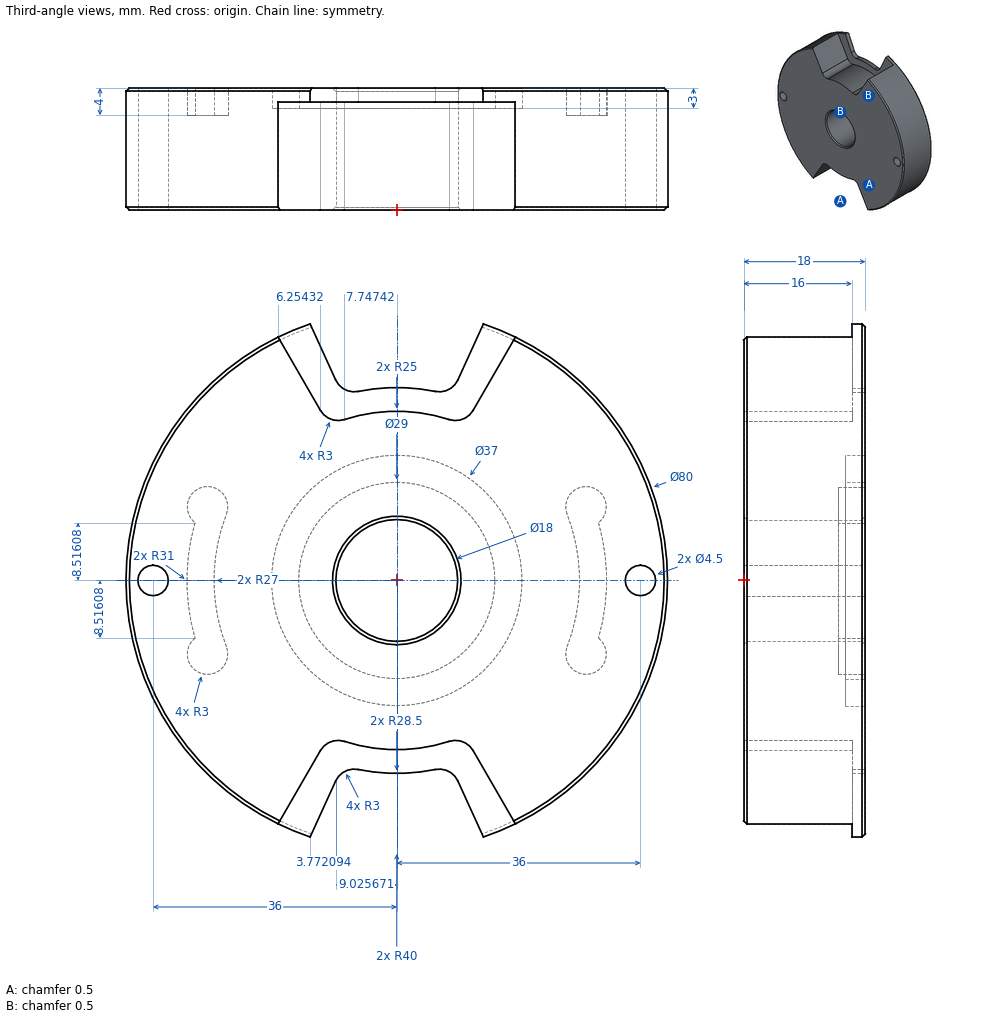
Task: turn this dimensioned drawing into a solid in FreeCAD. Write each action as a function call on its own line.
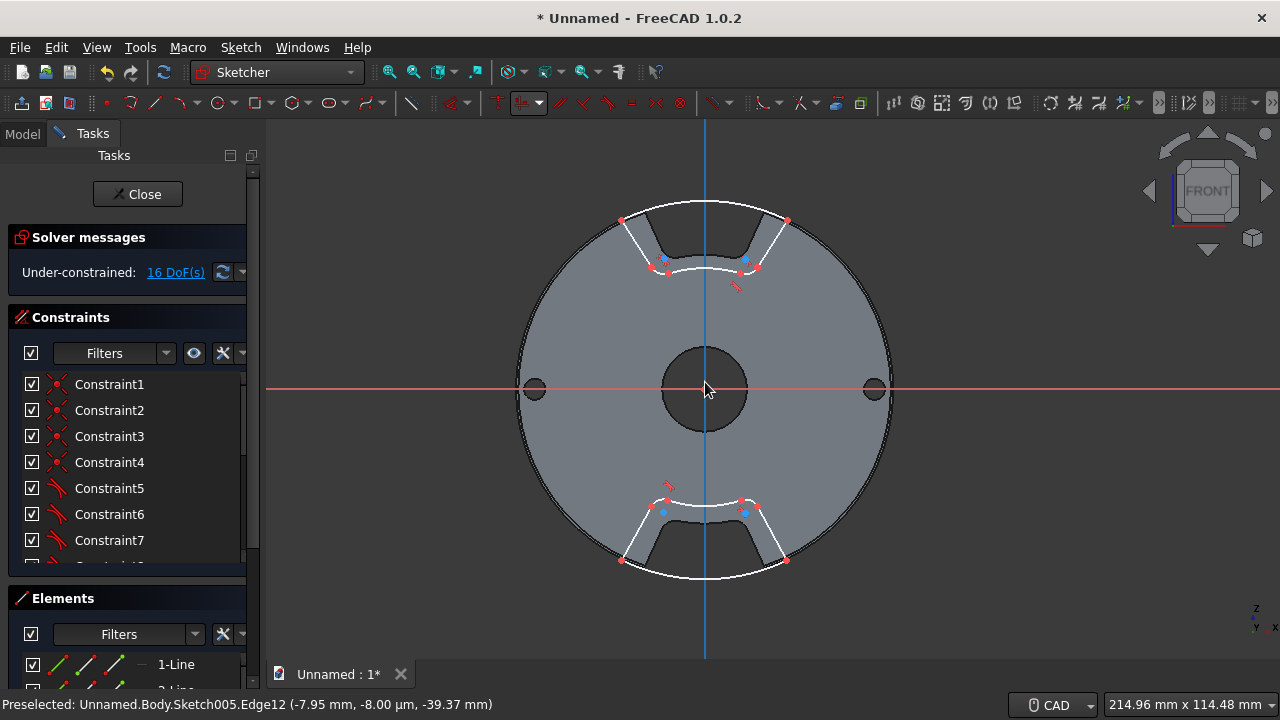
scroll(656, 271, up, 5)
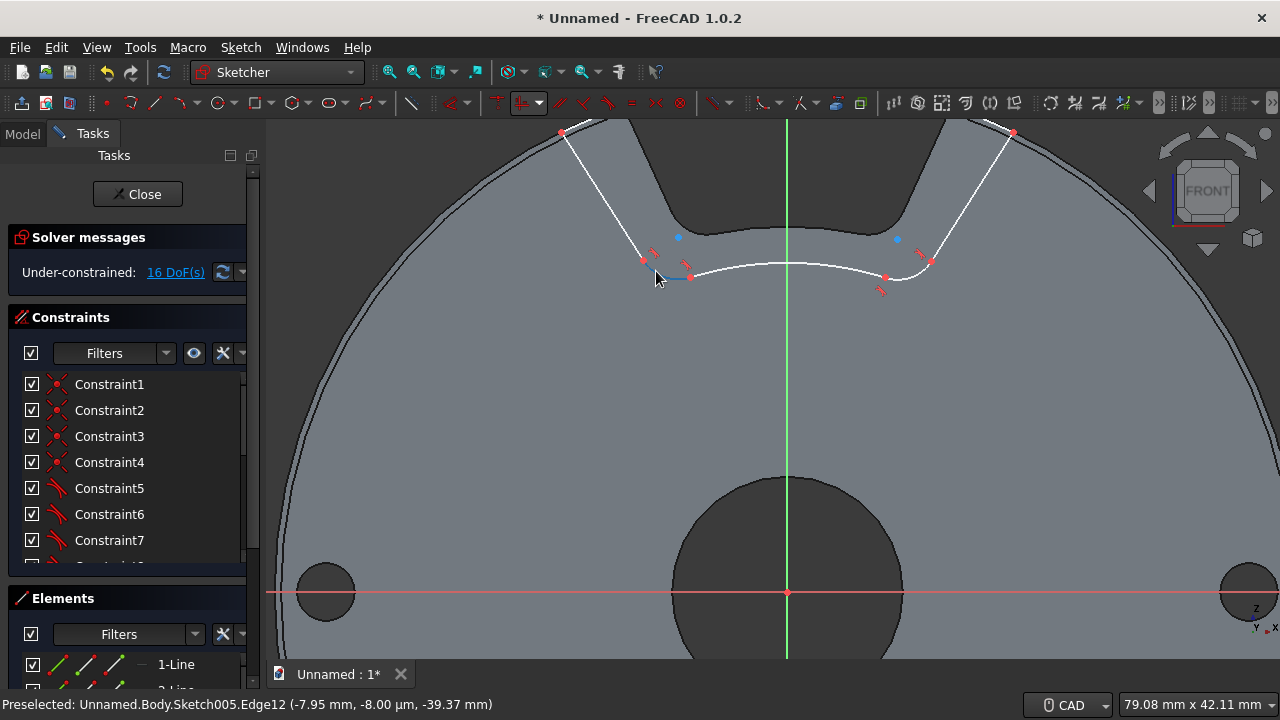
click(654, 272)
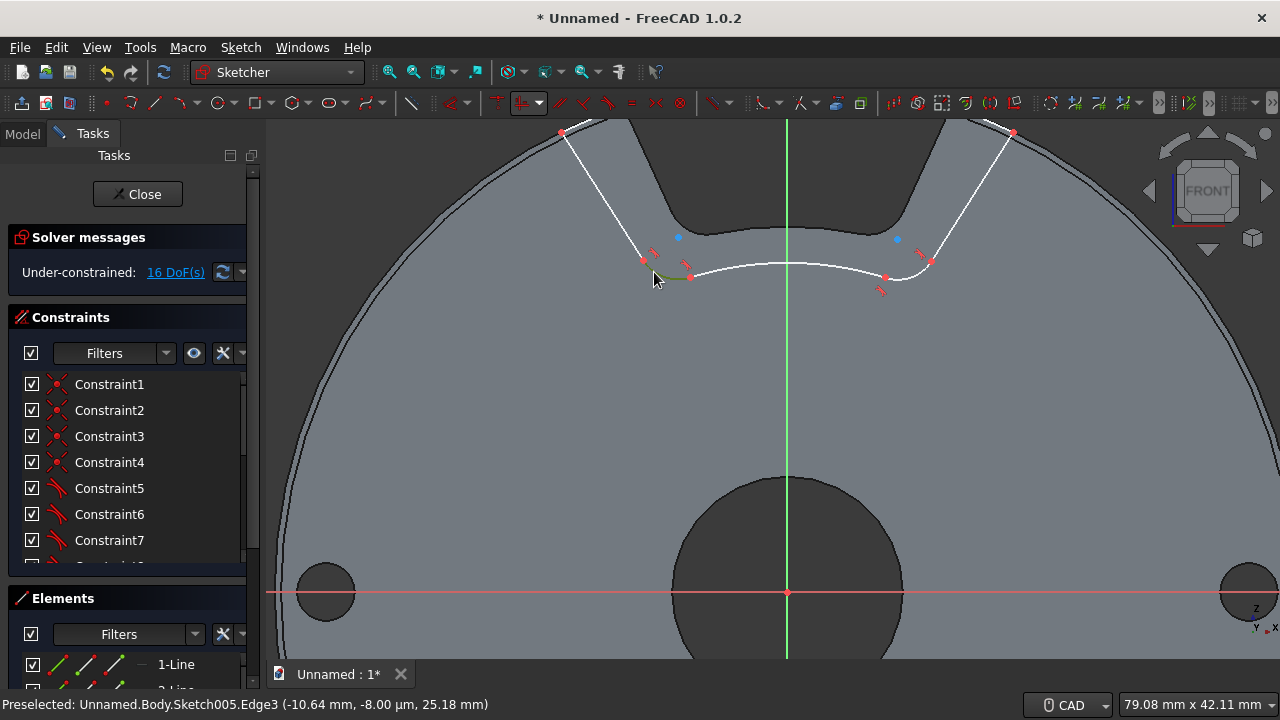
click(901, 280)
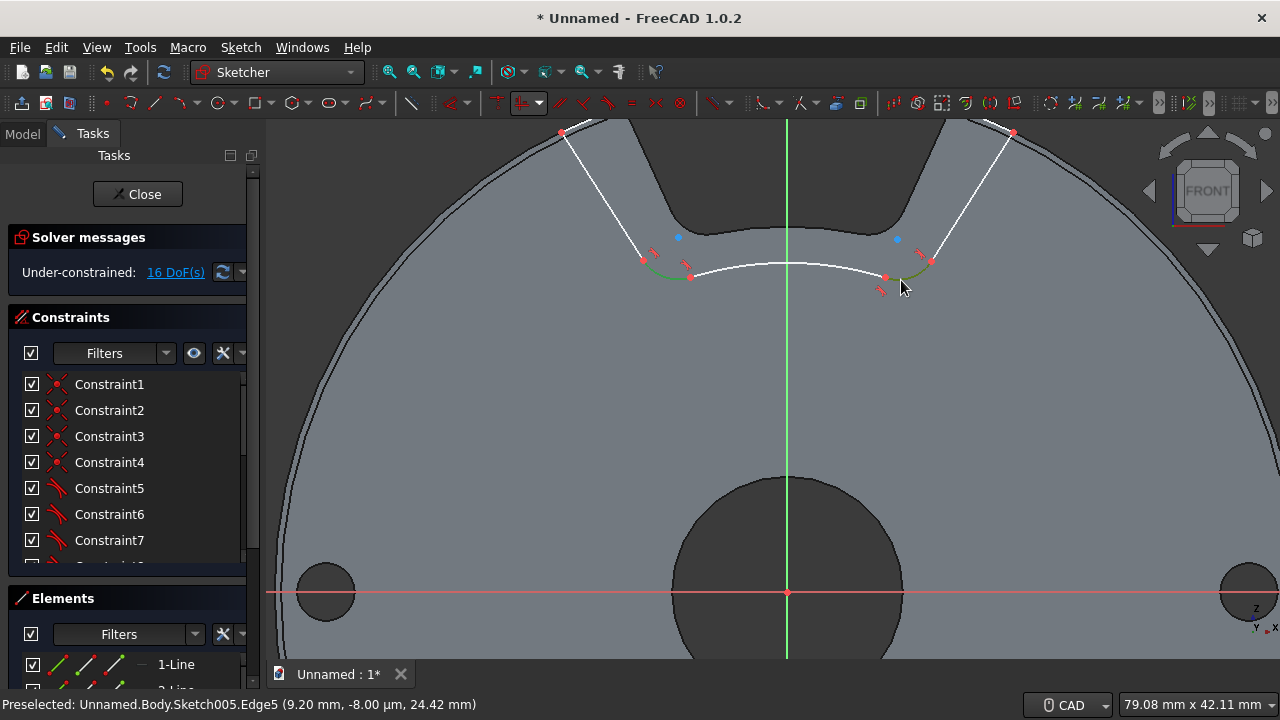
scroll(656, 271, down, 5)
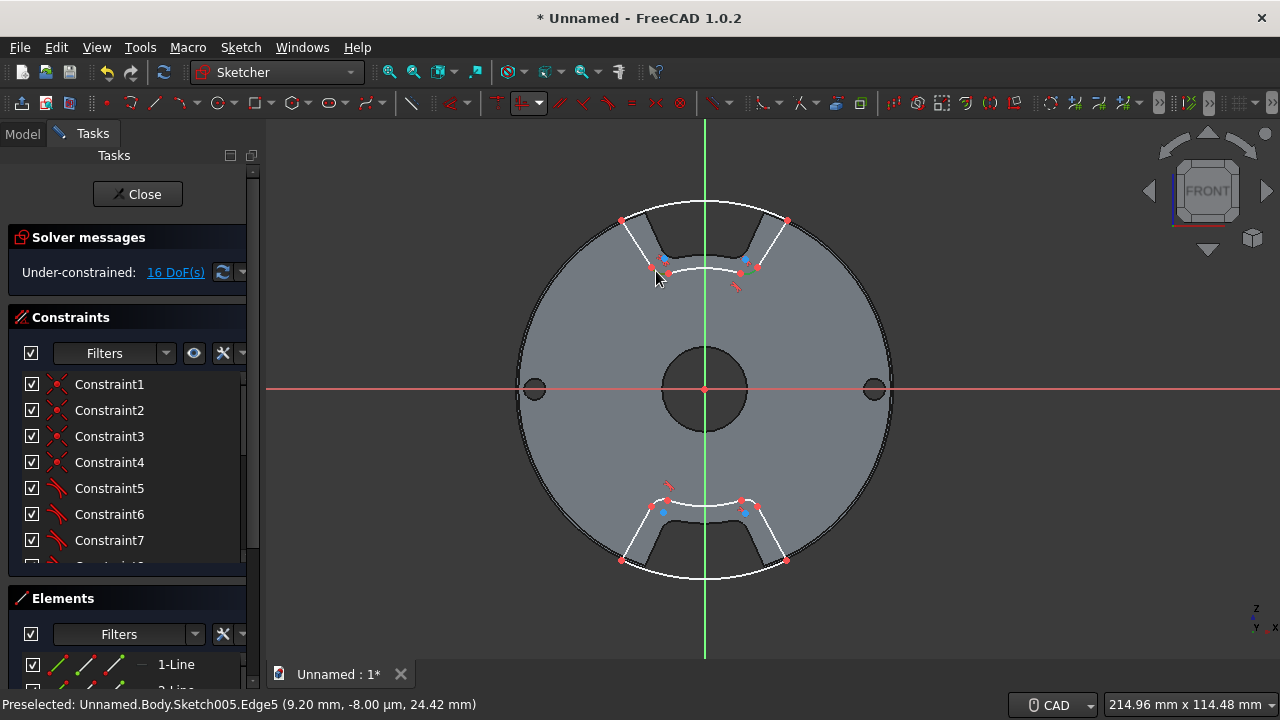
scroll(754, 502, up, 5)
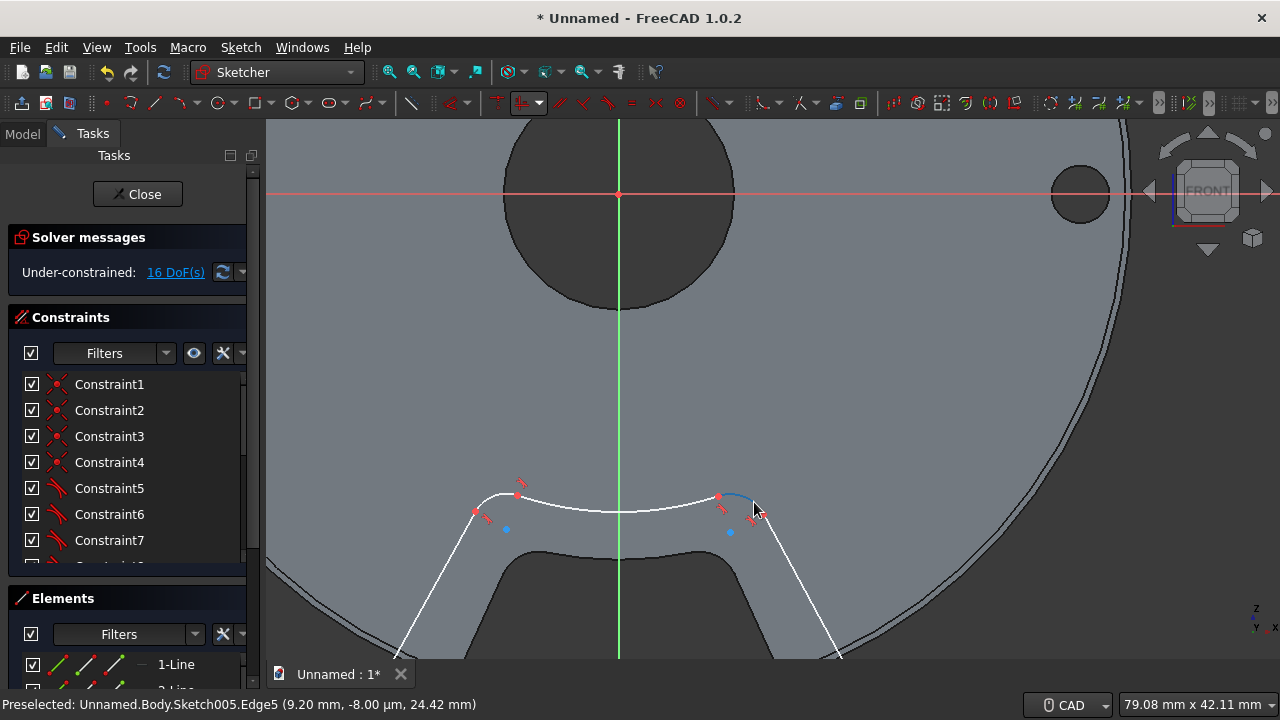
click(753, 502)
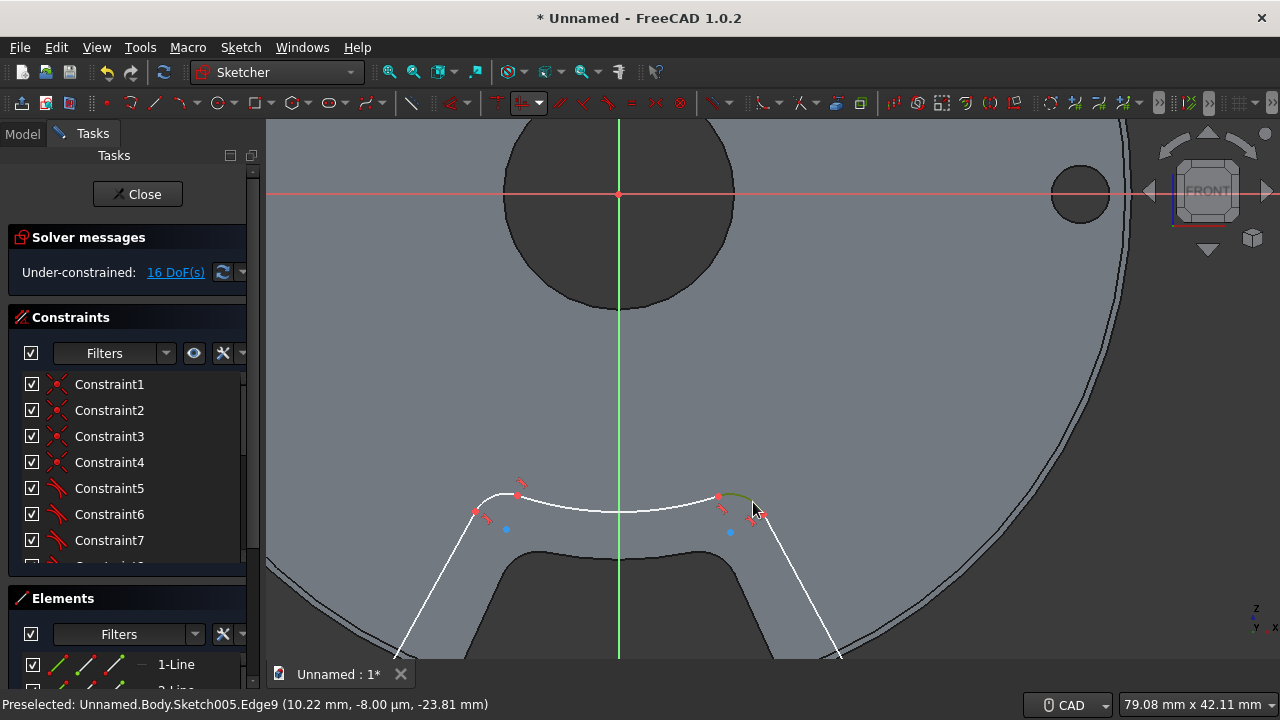
click(503, 494)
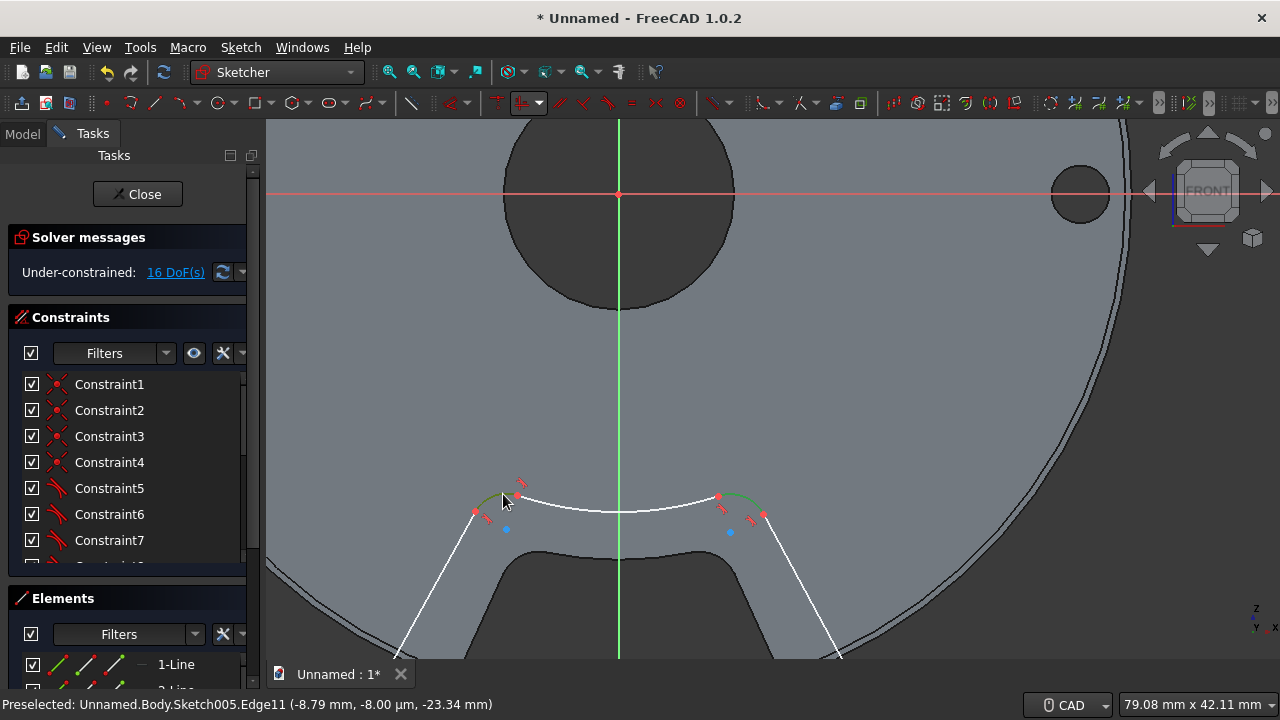
click(632, 104)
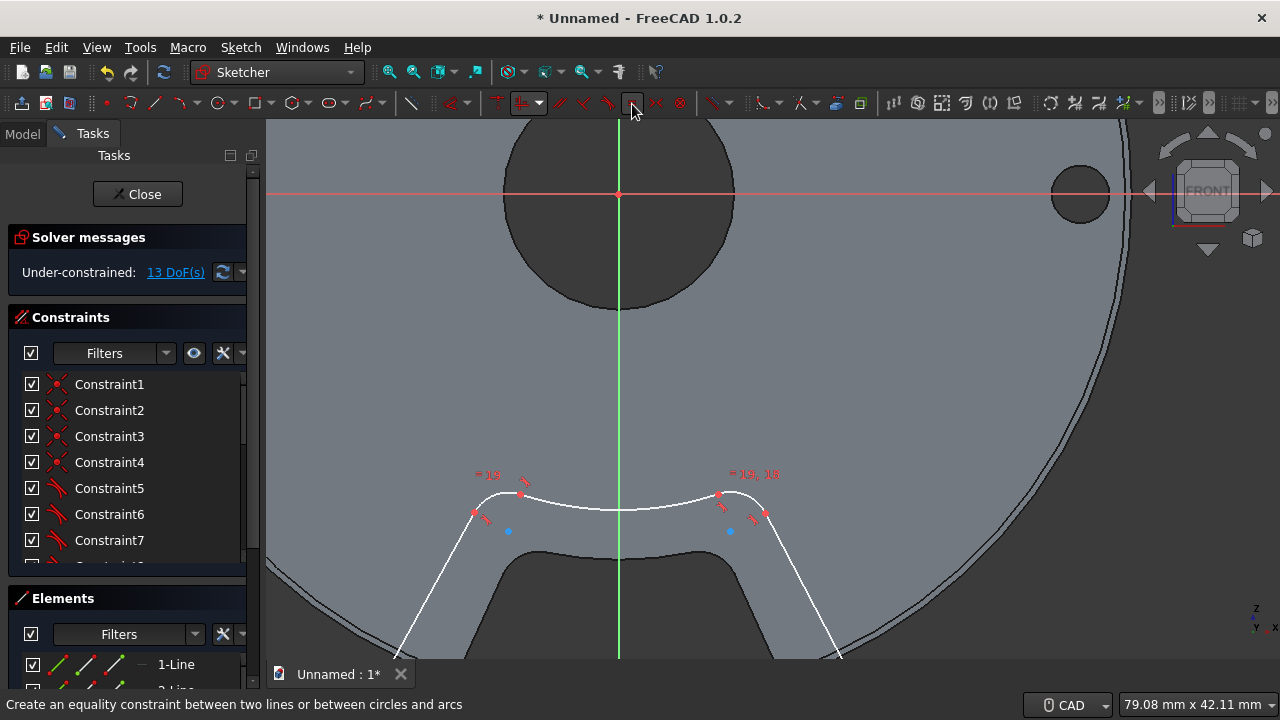
scroll(754, 502, down, 5)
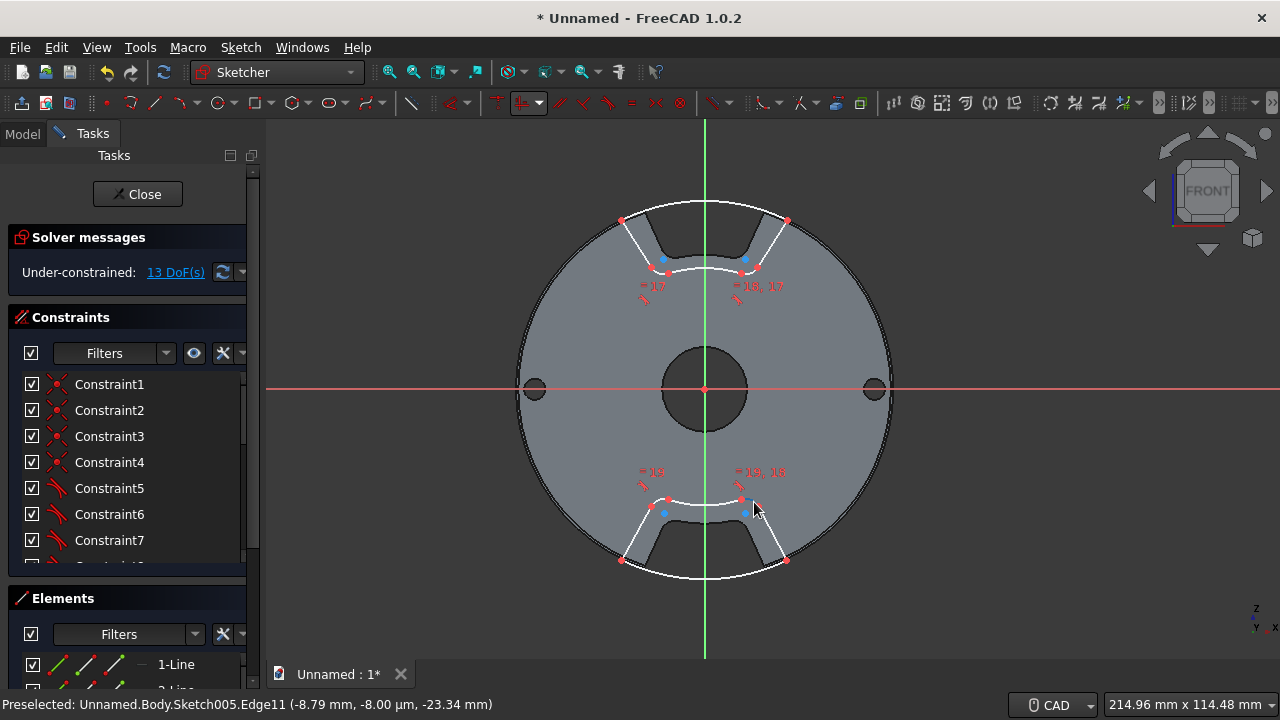
click(719, 269)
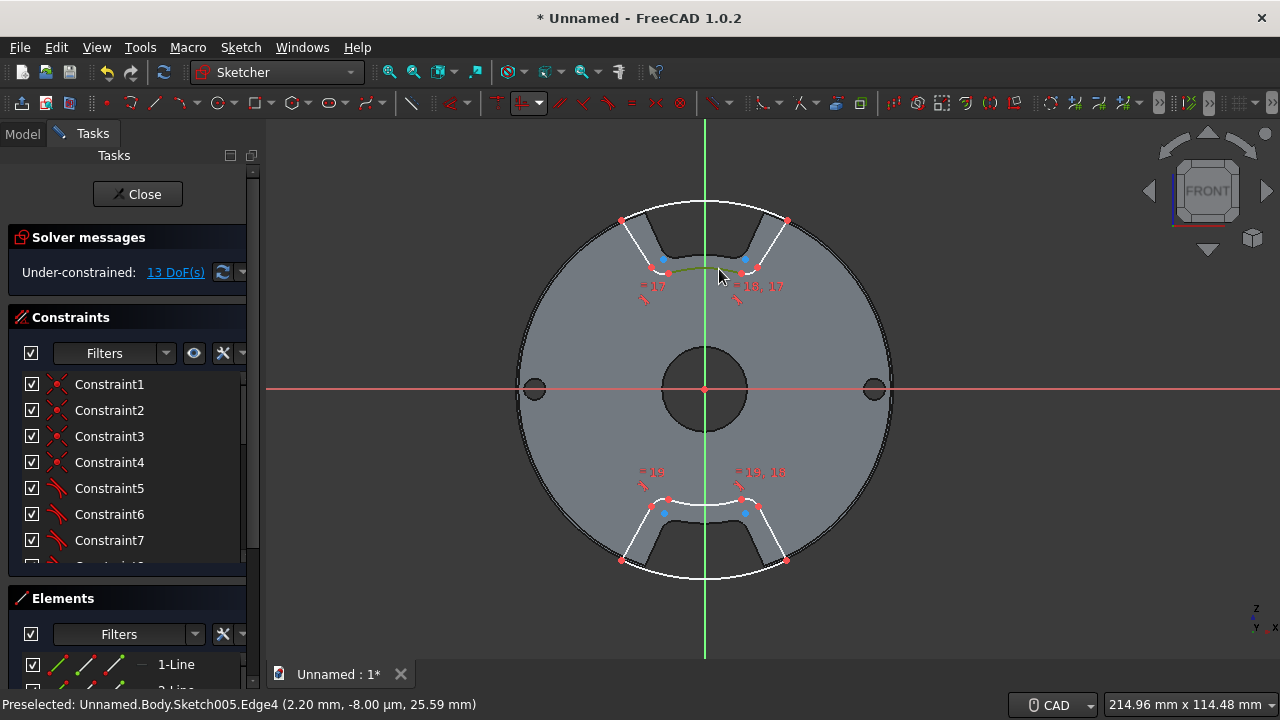
click(690, 505)